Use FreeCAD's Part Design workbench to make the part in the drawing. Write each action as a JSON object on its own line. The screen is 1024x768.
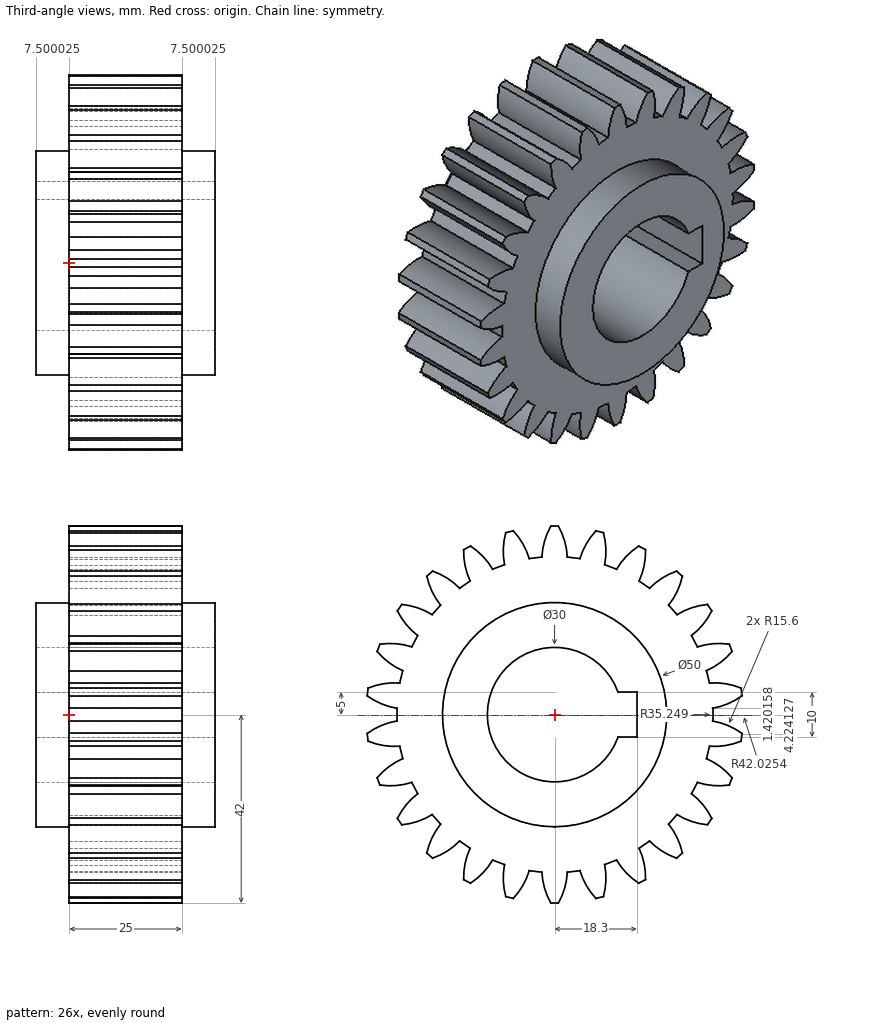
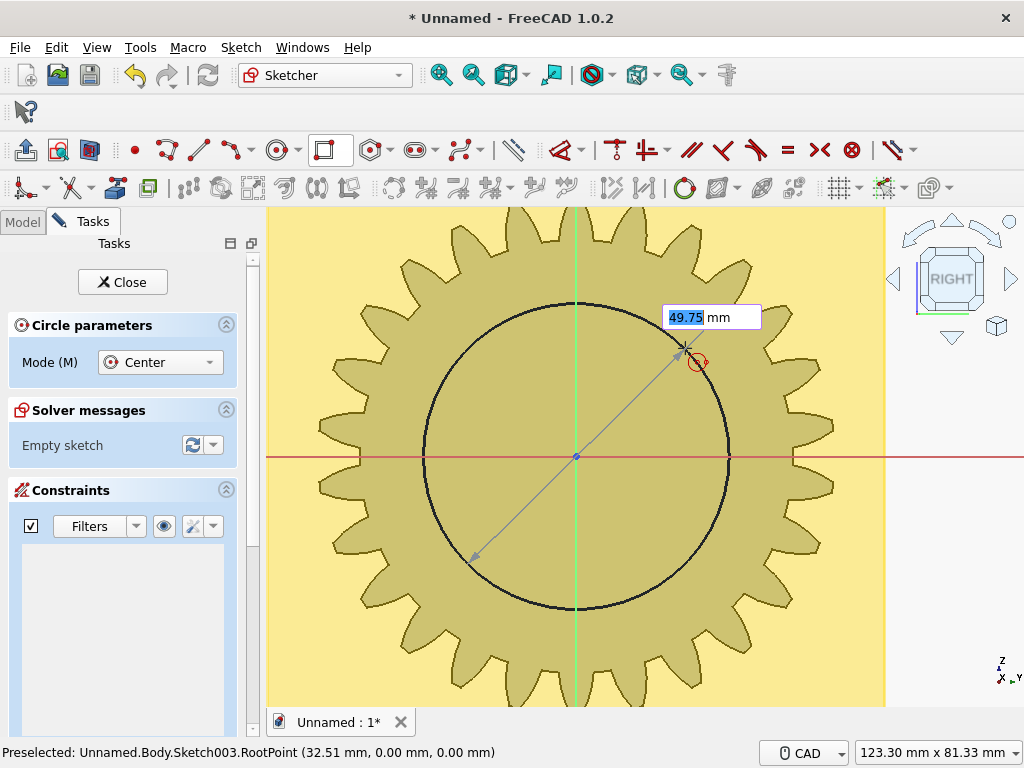
{"action": "type", "text": "50"}
{"action": "key", "text": "Return"}
{"action": "key", "text": "Escape"}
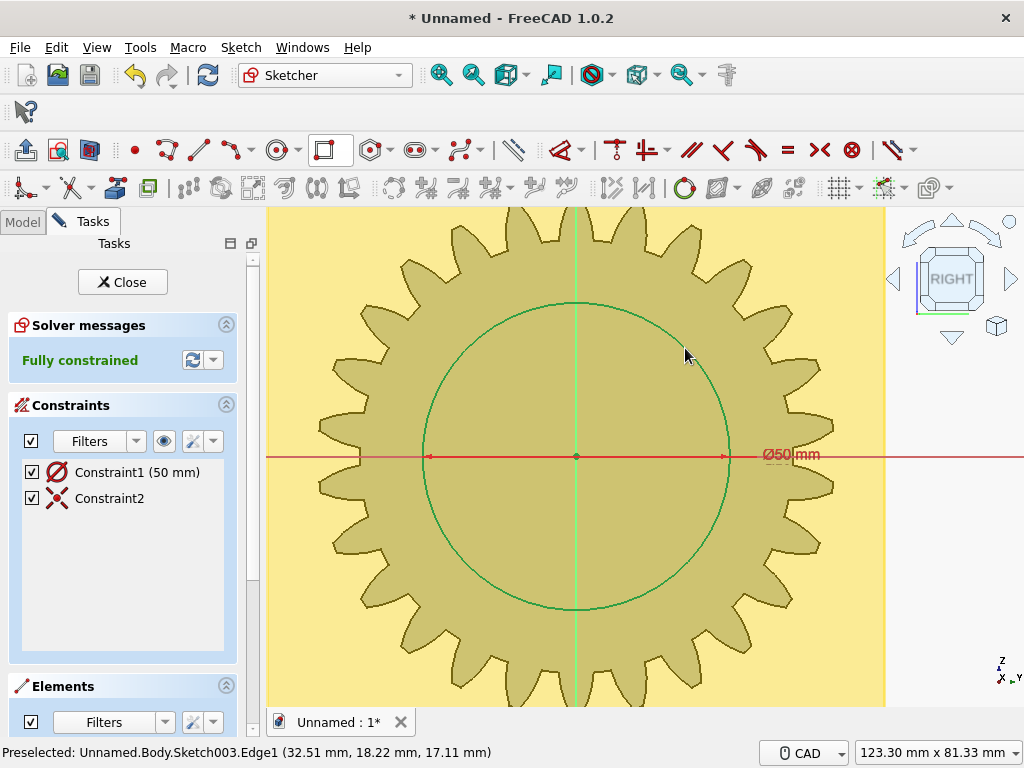
{"action": "left_click", "coordinate": [123, 282]}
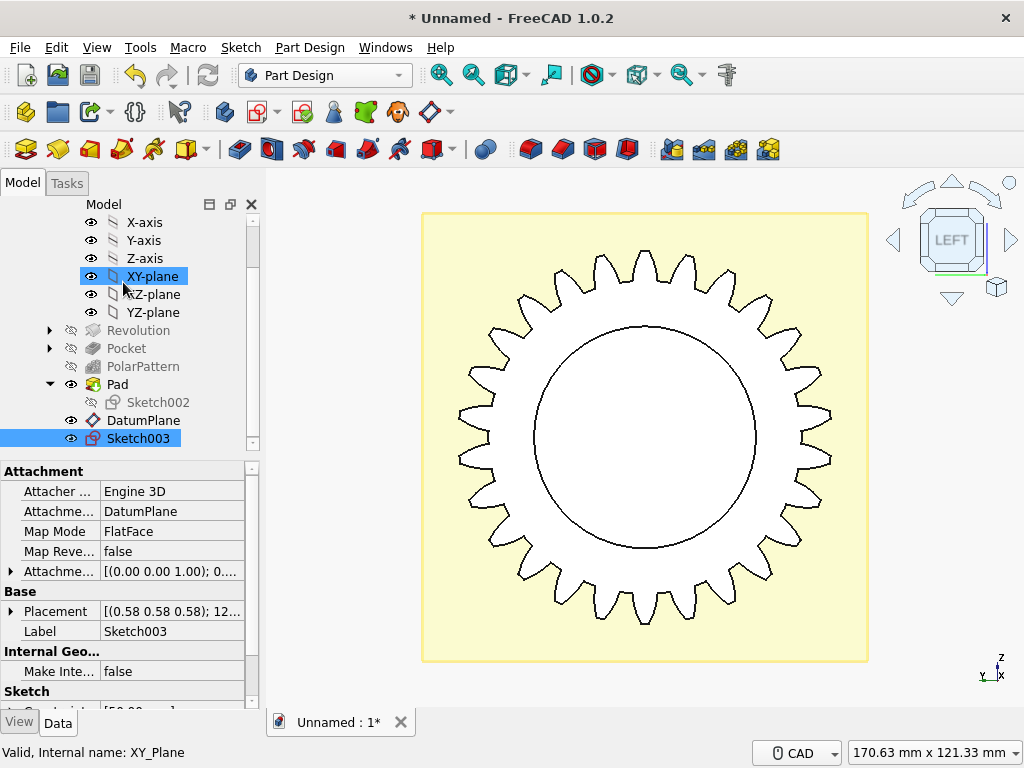
{"action": "left_click", "coordinate": [26, 150]}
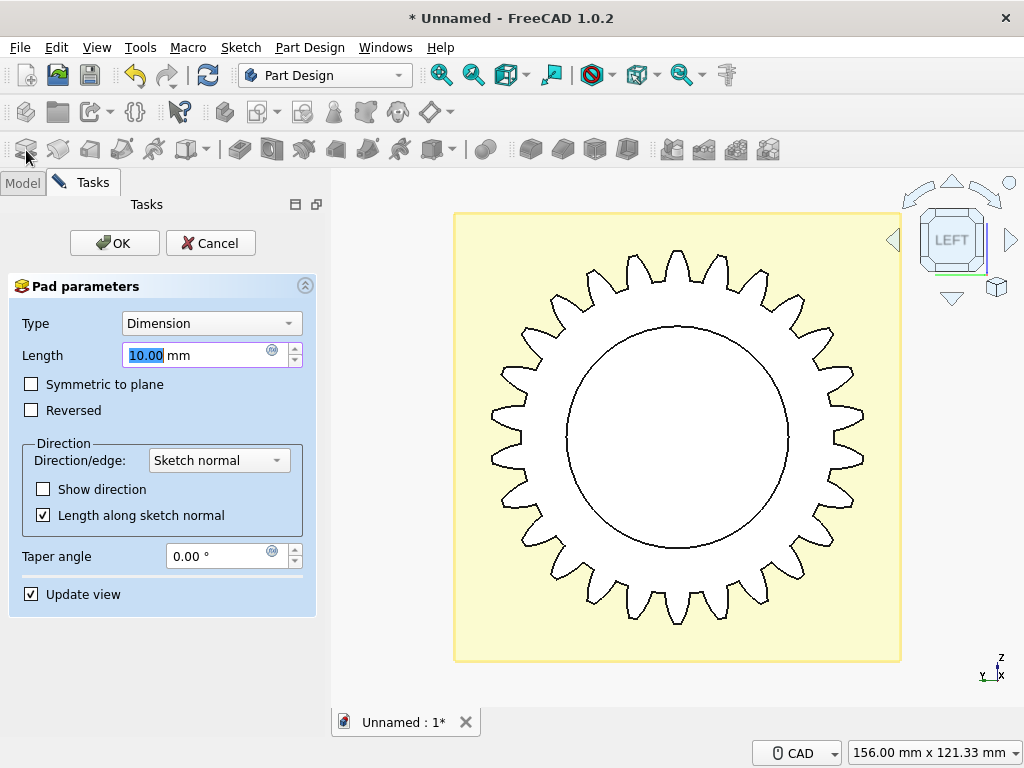
{"action": "type", "text": "7.500025"}
{"action": "key", "text": "Tab"}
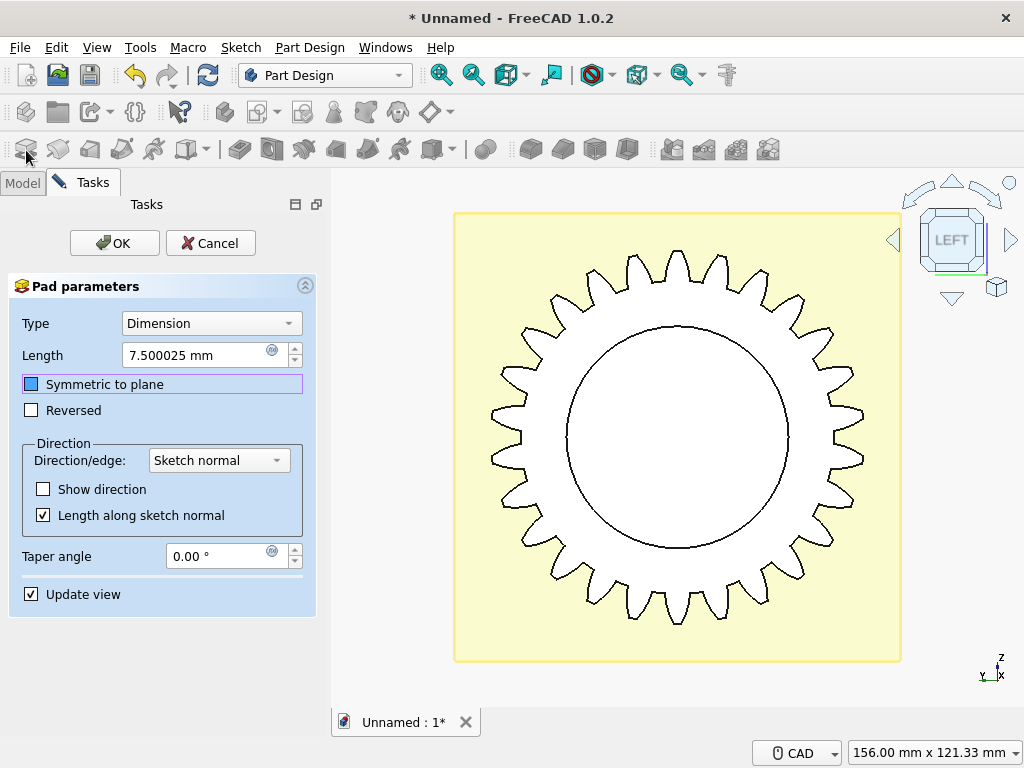
{"action": "left_click", "coordinate": [30, 410]}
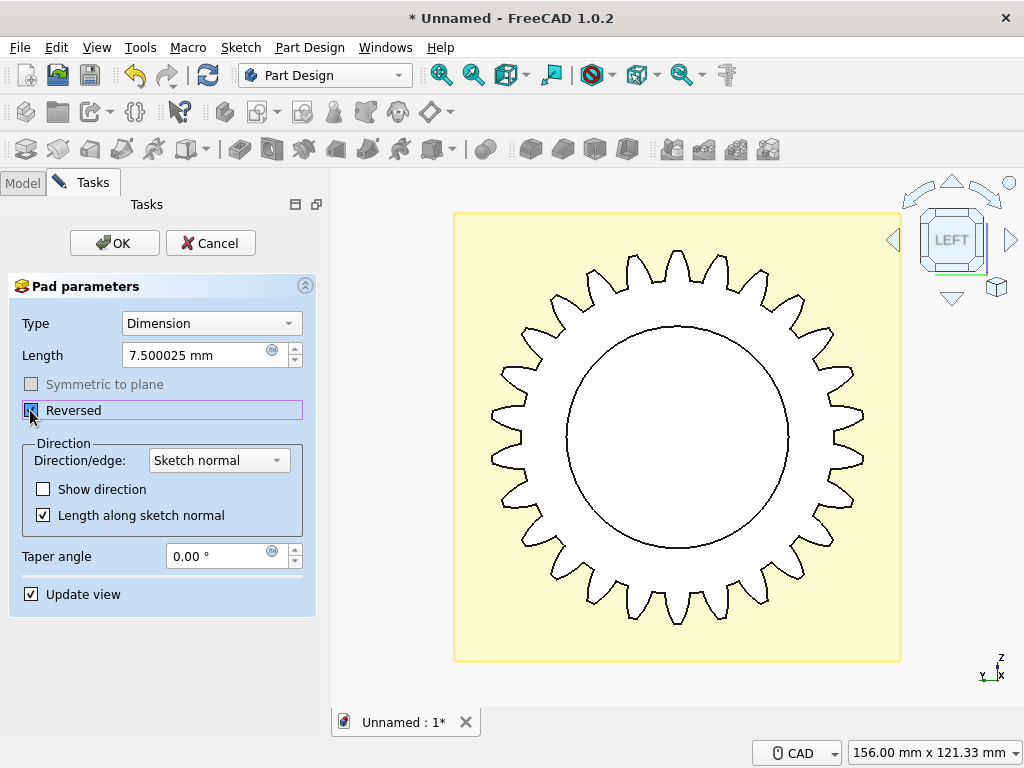
{"action": "left_click", "coordinate": [115, 243]}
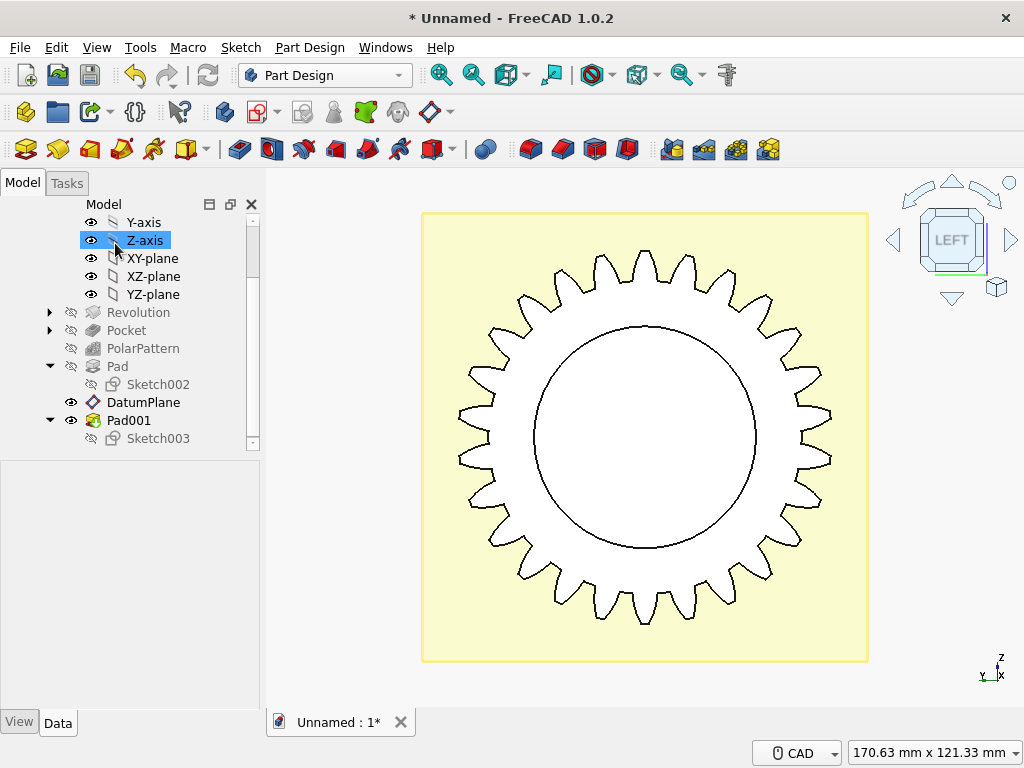
{"action": "left_click", "coordinate": [116, 402]}
{"action": "key", "text": "space"}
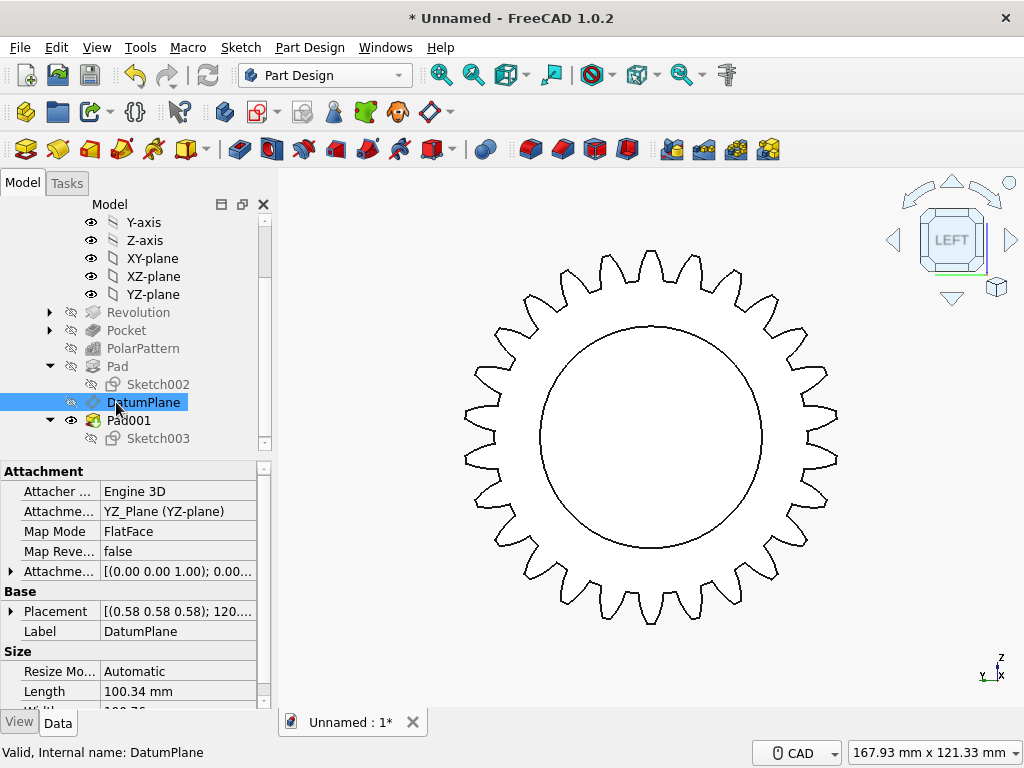
{"action": "left_click", "coordinate": [651, 276]}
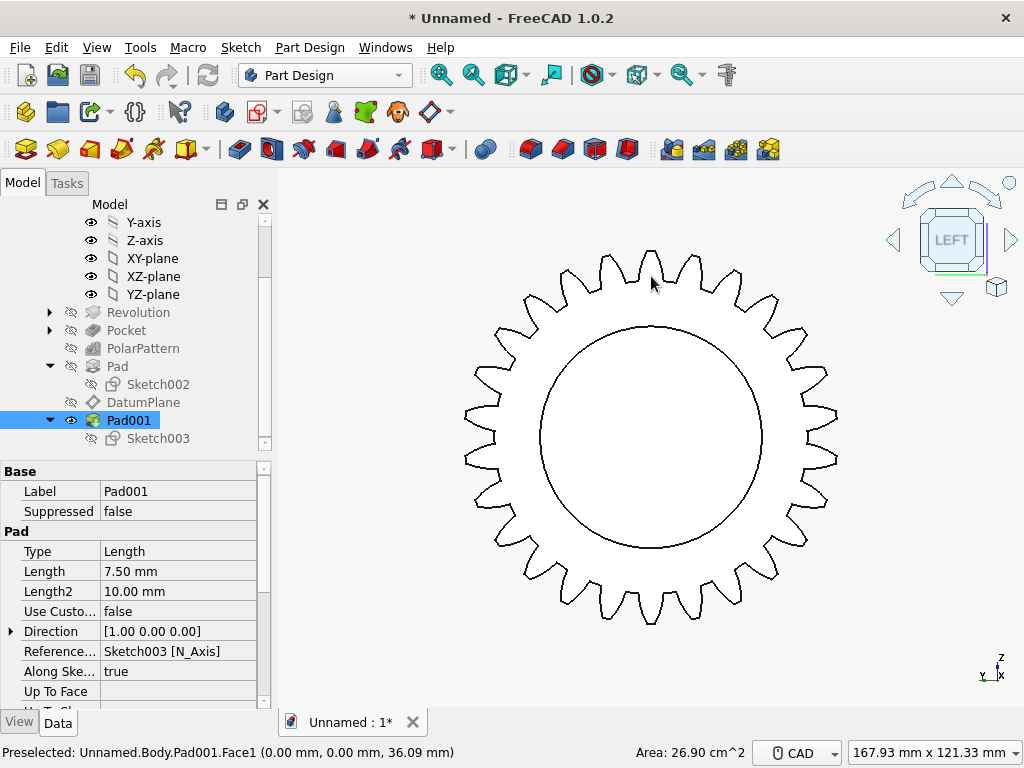
{"action": "left_click", "coordinate": [258, 112]}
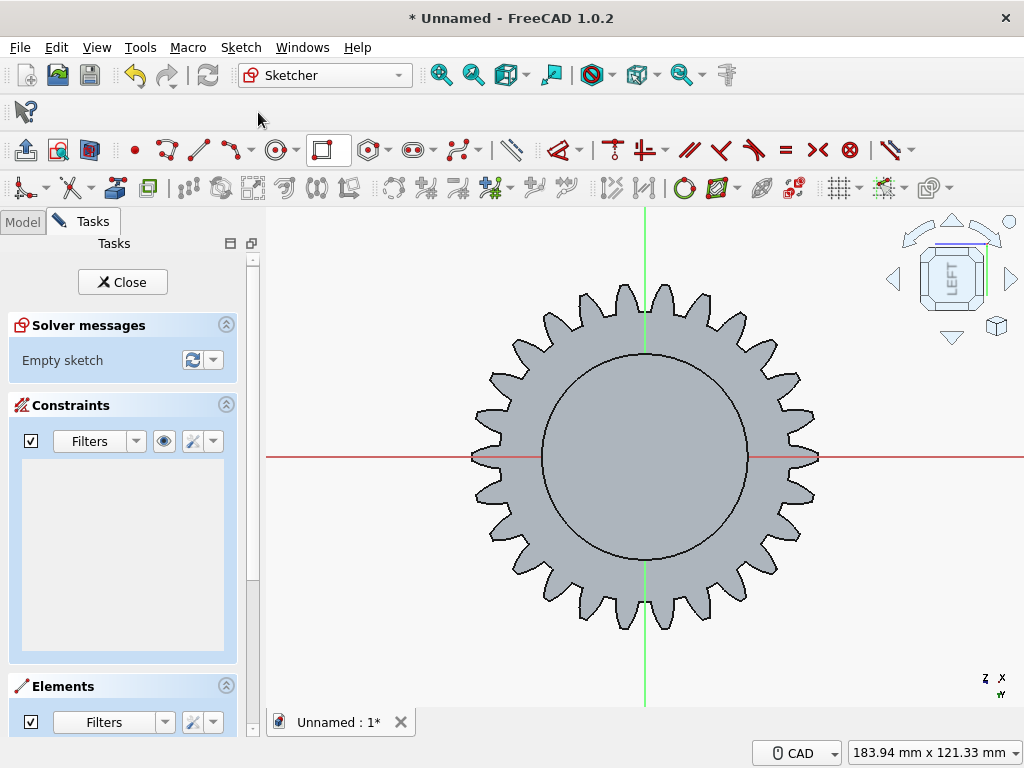
{"action": "scroll", "coordinate": [685, 457], "scroll_direction": "up", "scroll_amount": 5}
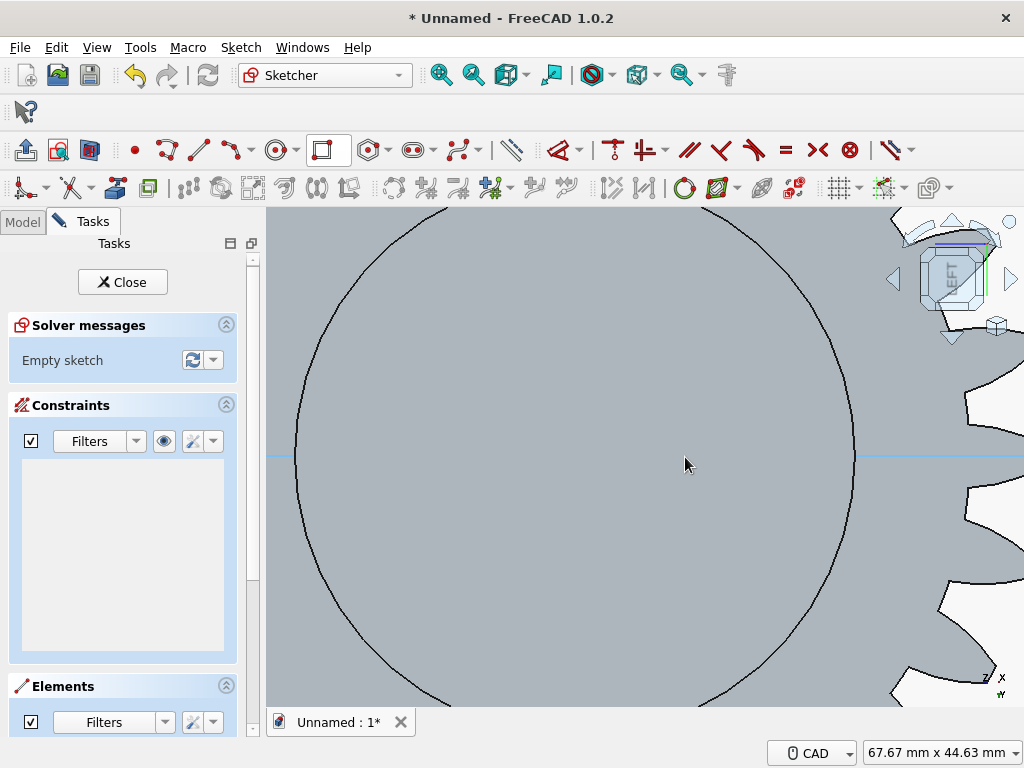
{"action": "left_click", "coordinate": [276, 150]}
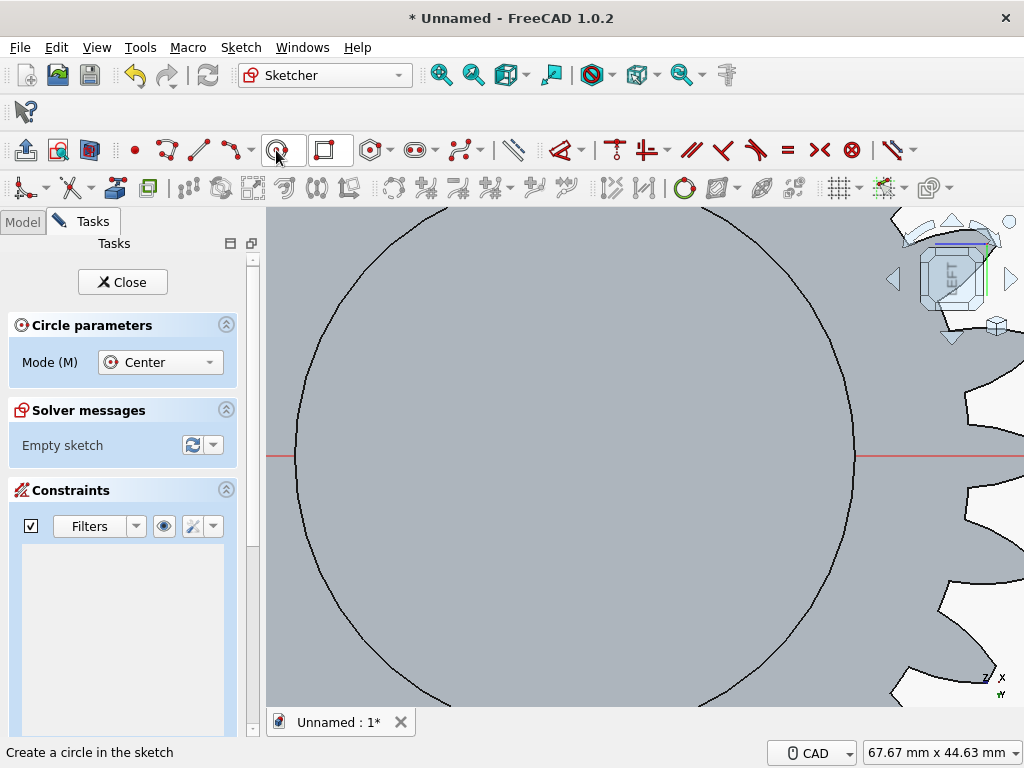
{"action": "left_click", "coordinate": [575, 456]}
{"action": "mouse_move", "coordinate": [694, 337]}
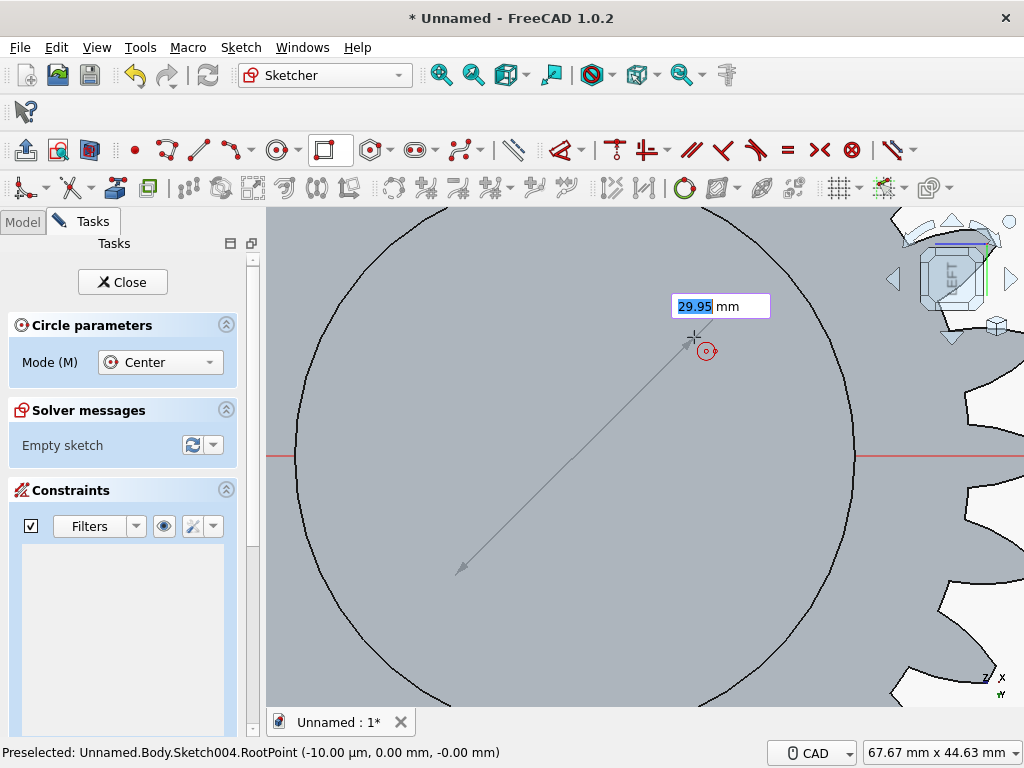
{"action": "type", "text": "30"}
{"action": "key", "text": "Return"}
{"action": "key", "text": "Escape"}